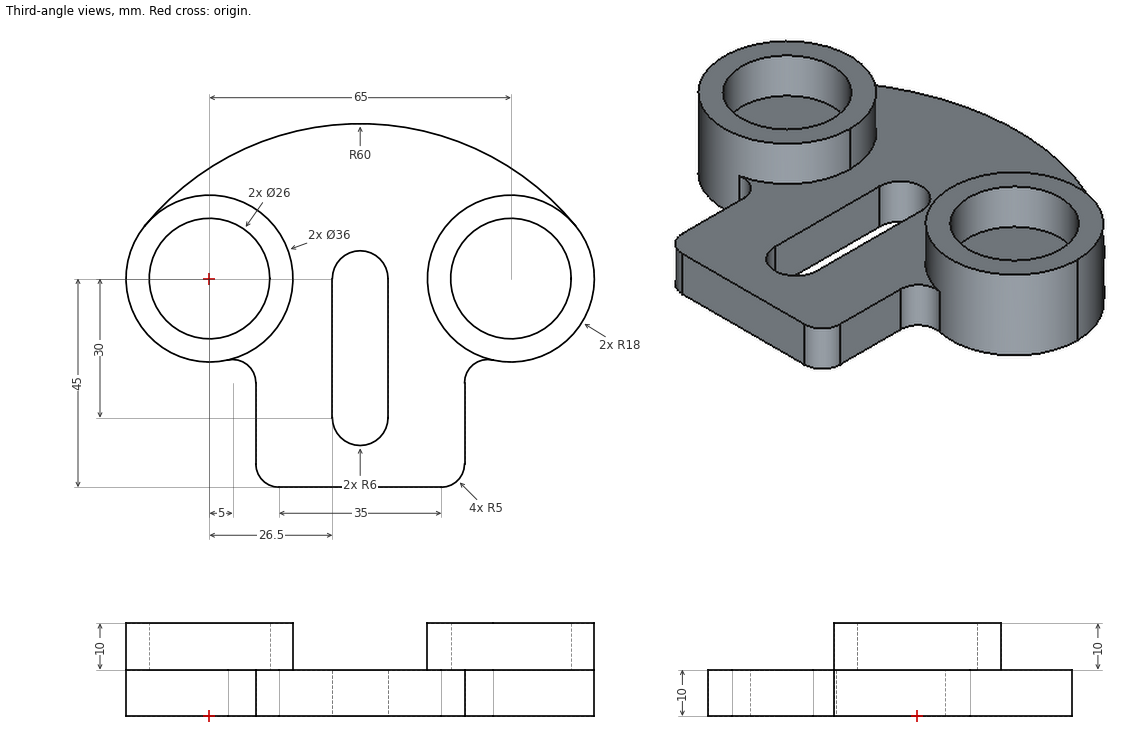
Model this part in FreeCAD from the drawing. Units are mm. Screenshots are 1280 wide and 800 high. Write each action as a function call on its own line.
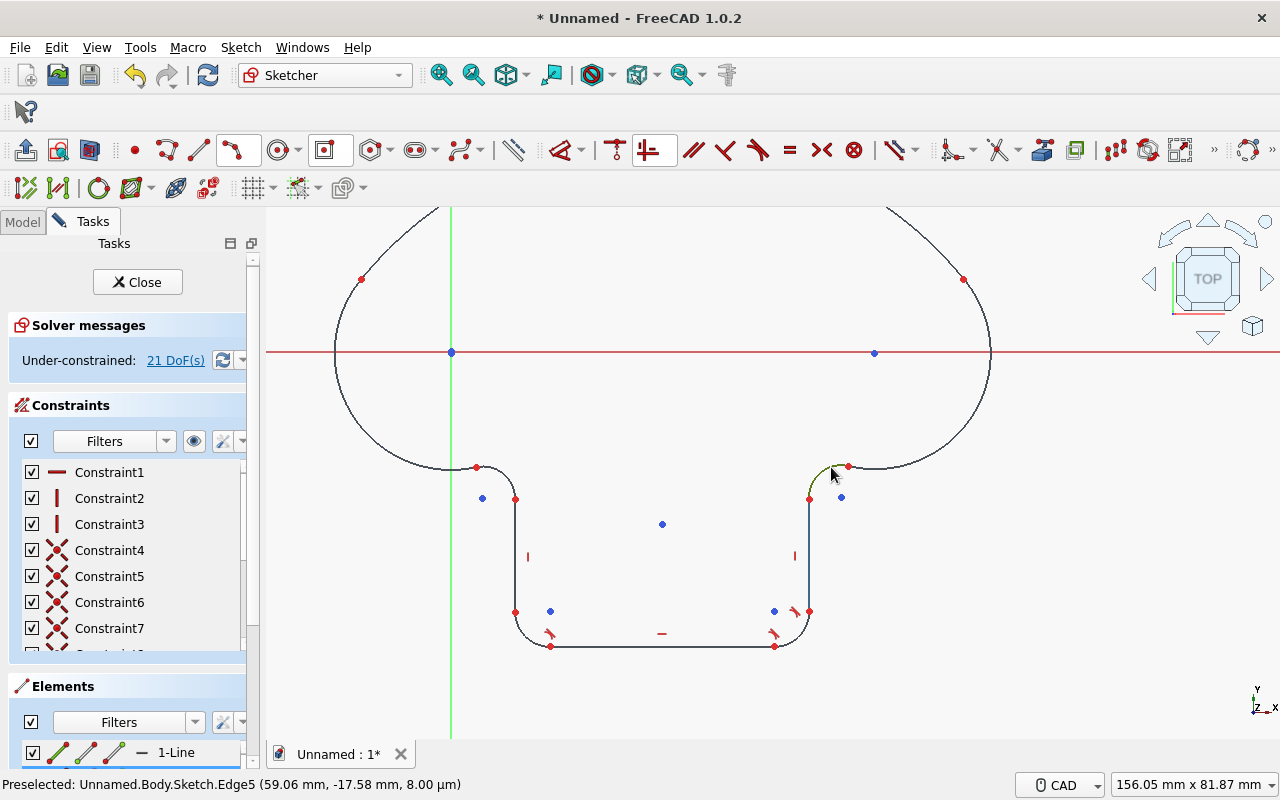
click(758, 150)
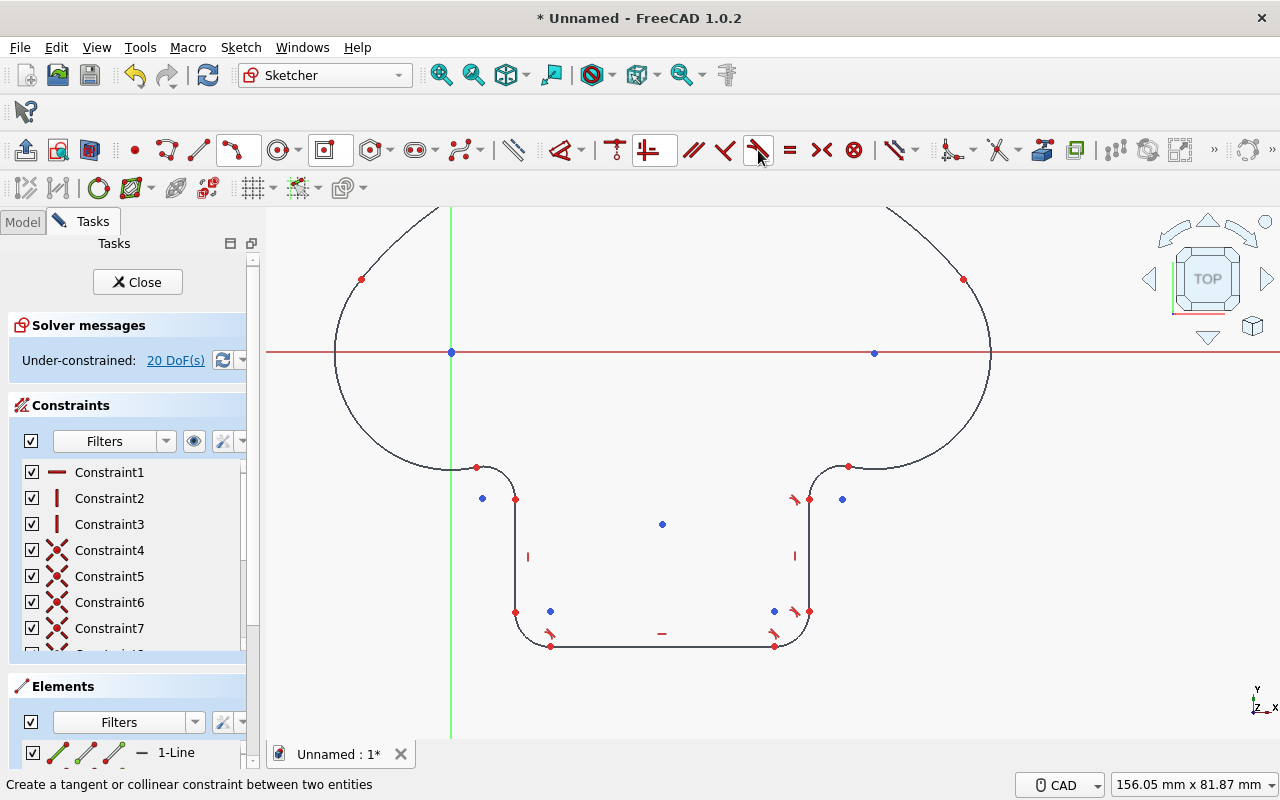
click(515, 534)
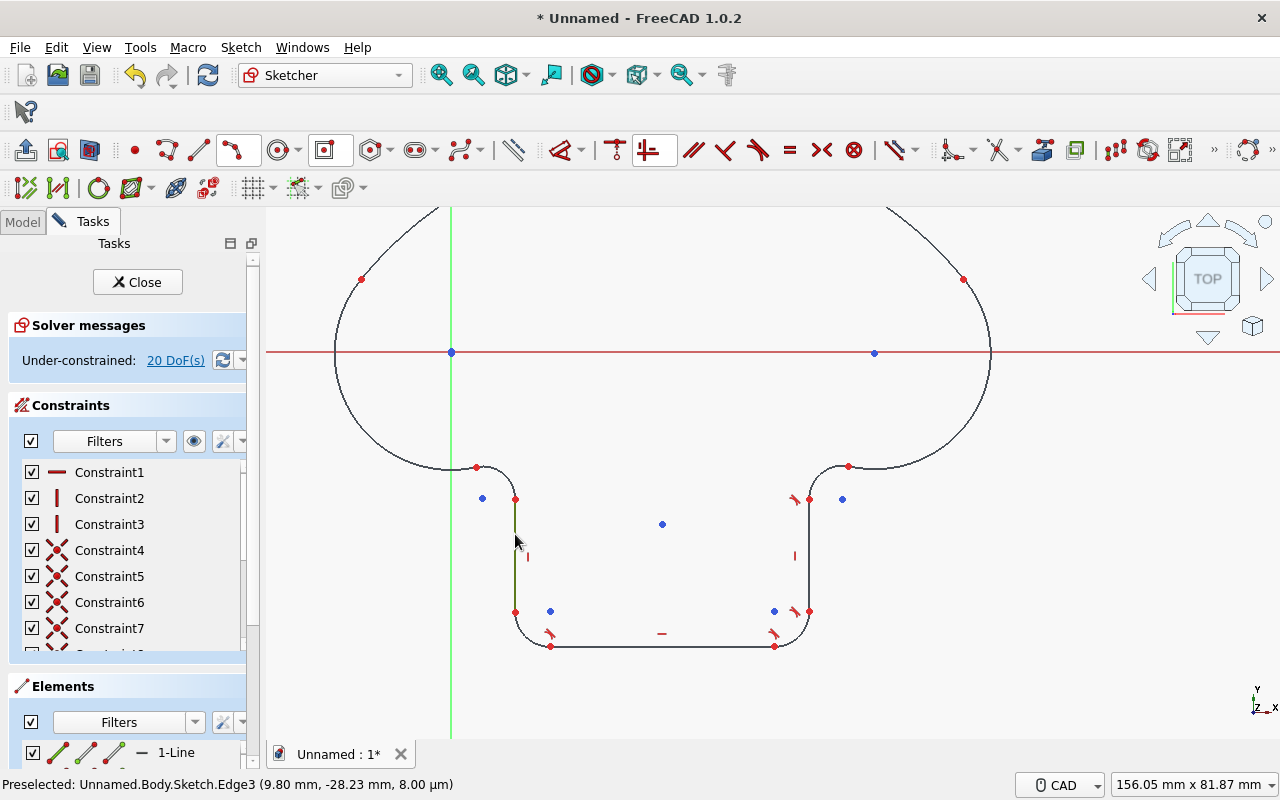
click(511, 483)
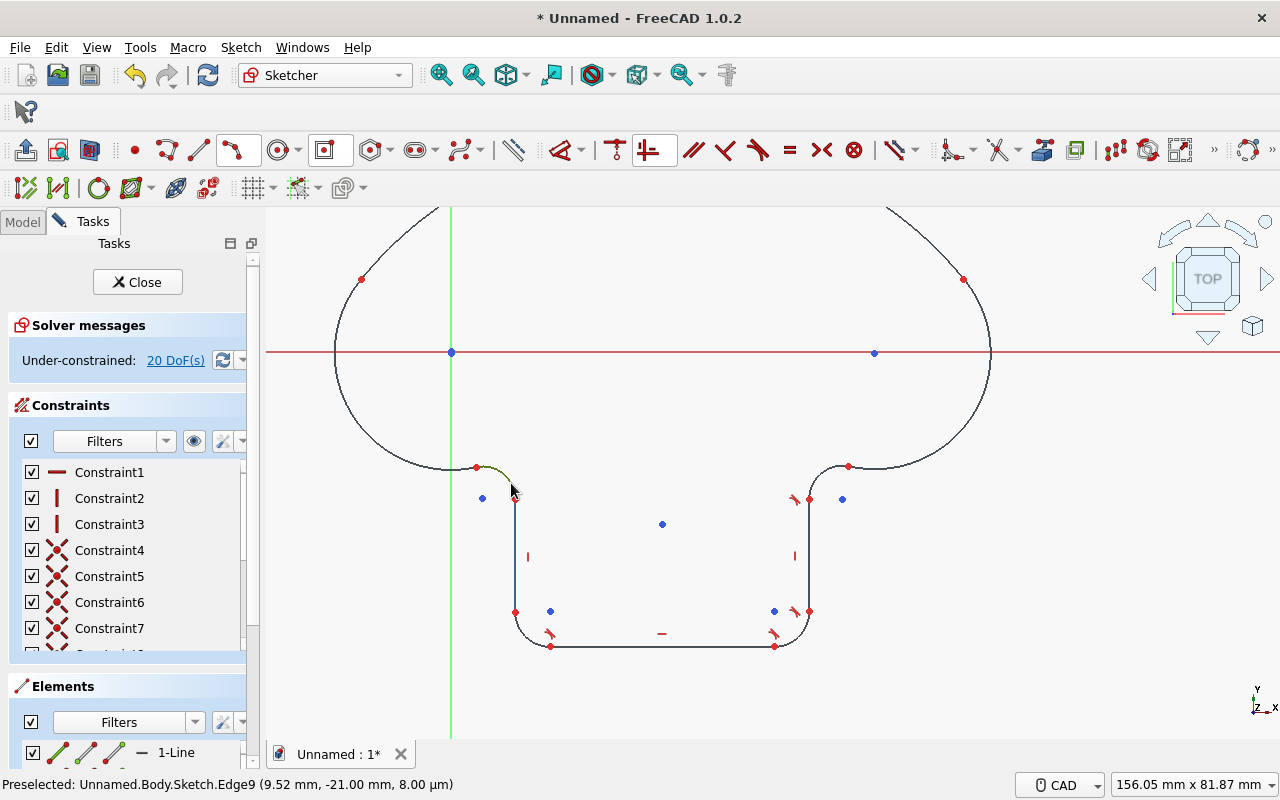
click(758, 150)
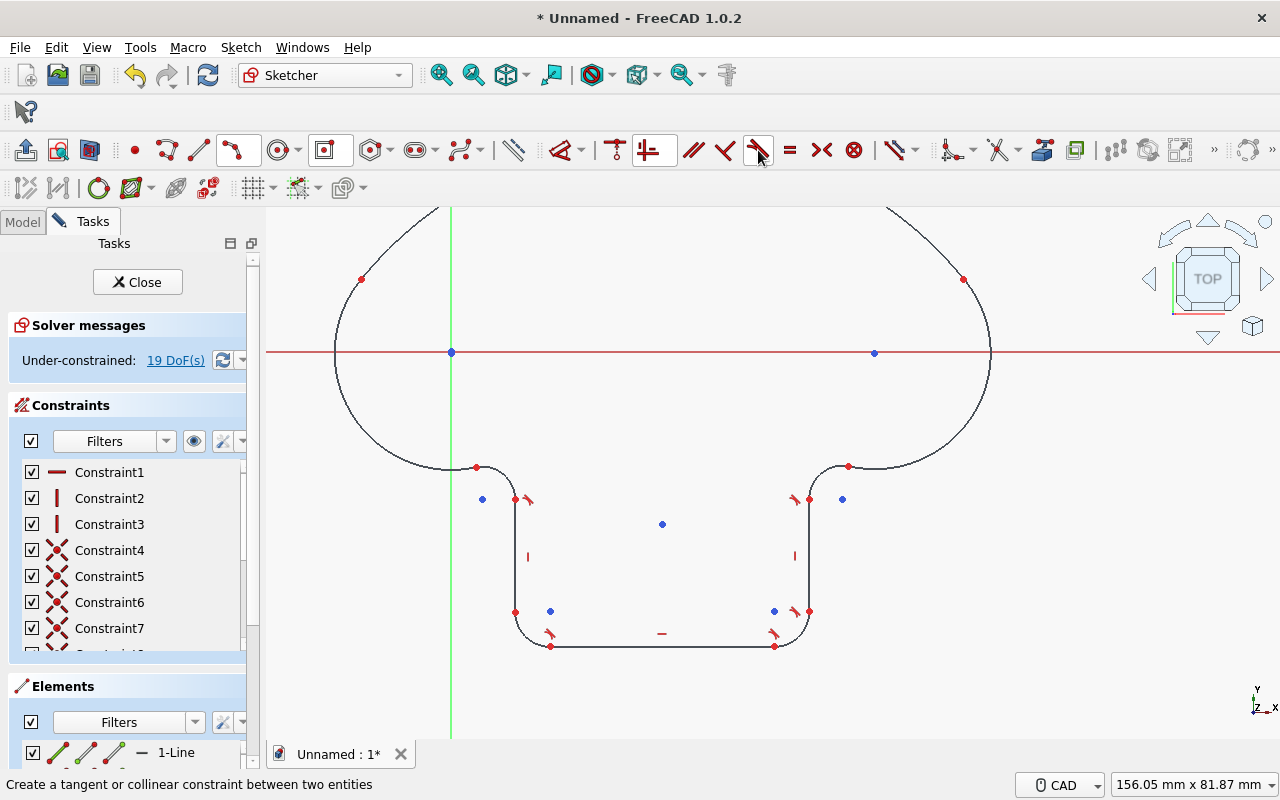
click(515, 534)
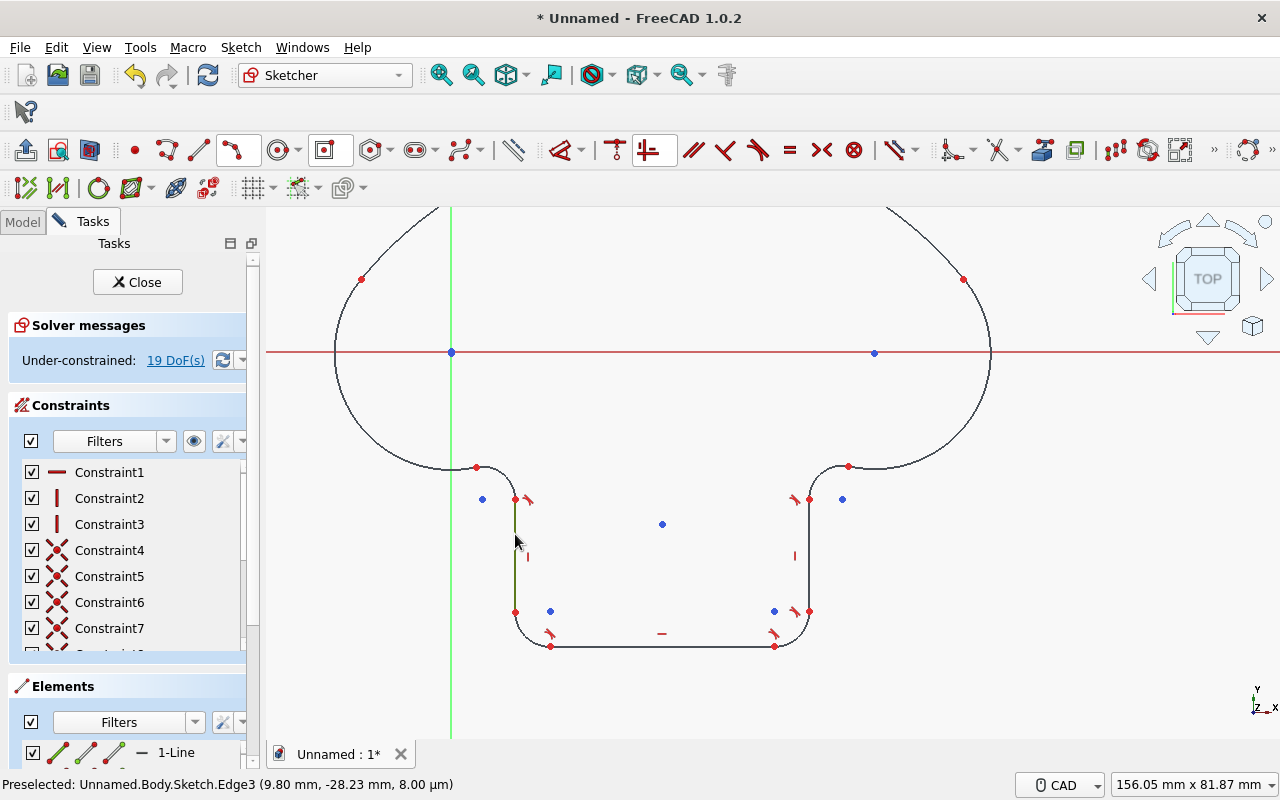
click(519, 628)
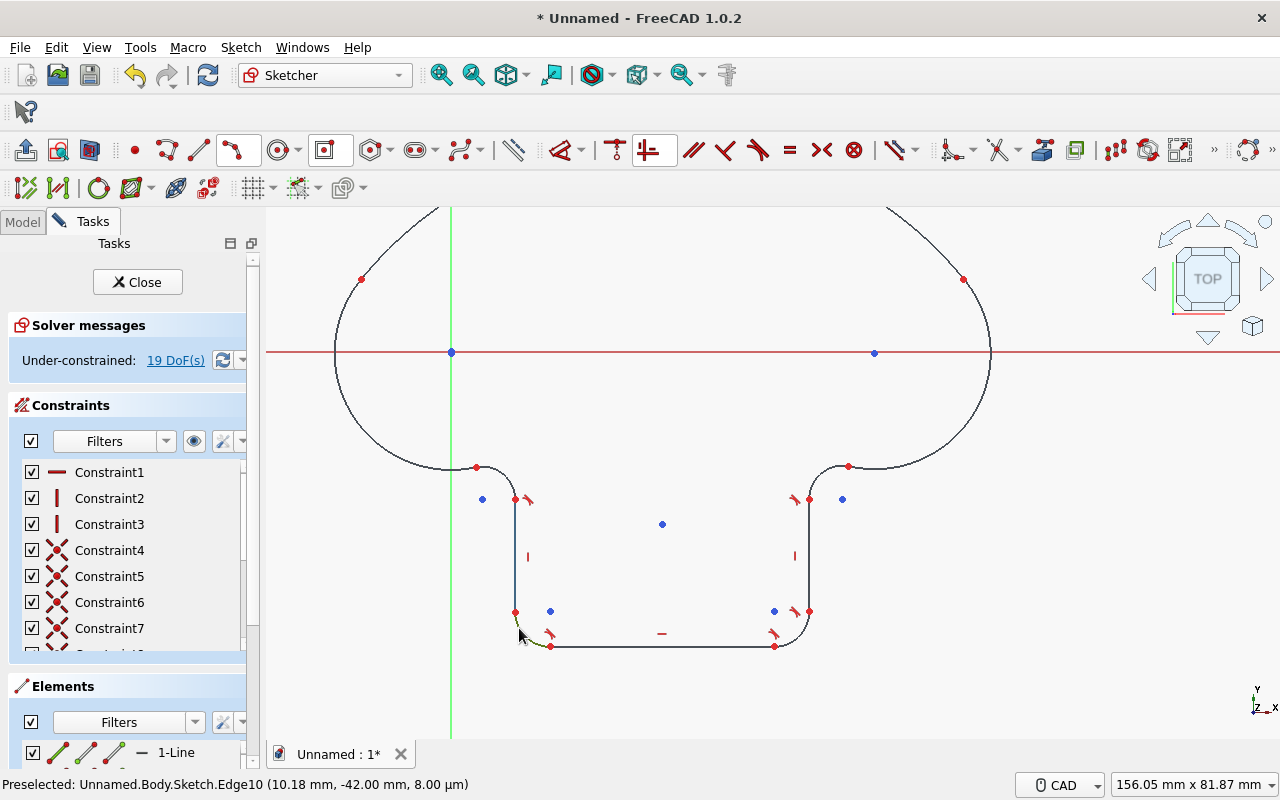
click(758, 150)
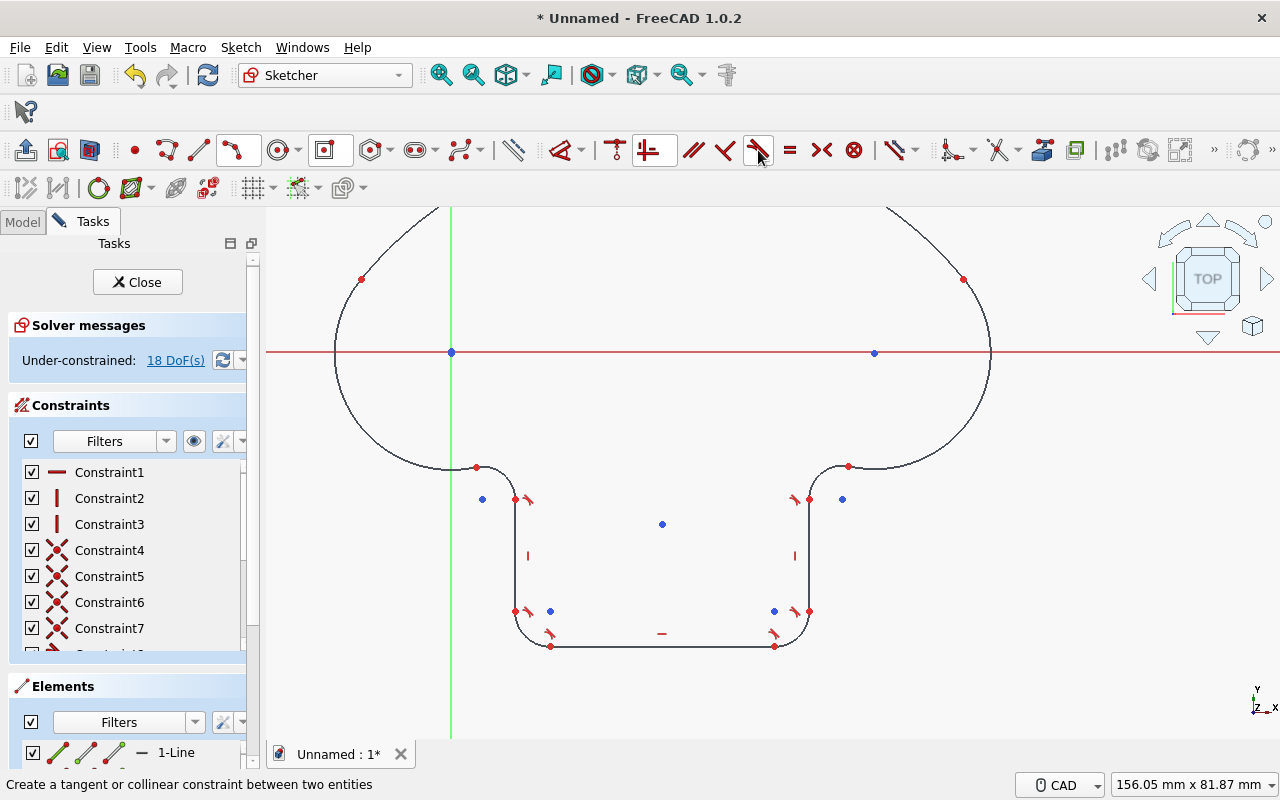
click(831, 468)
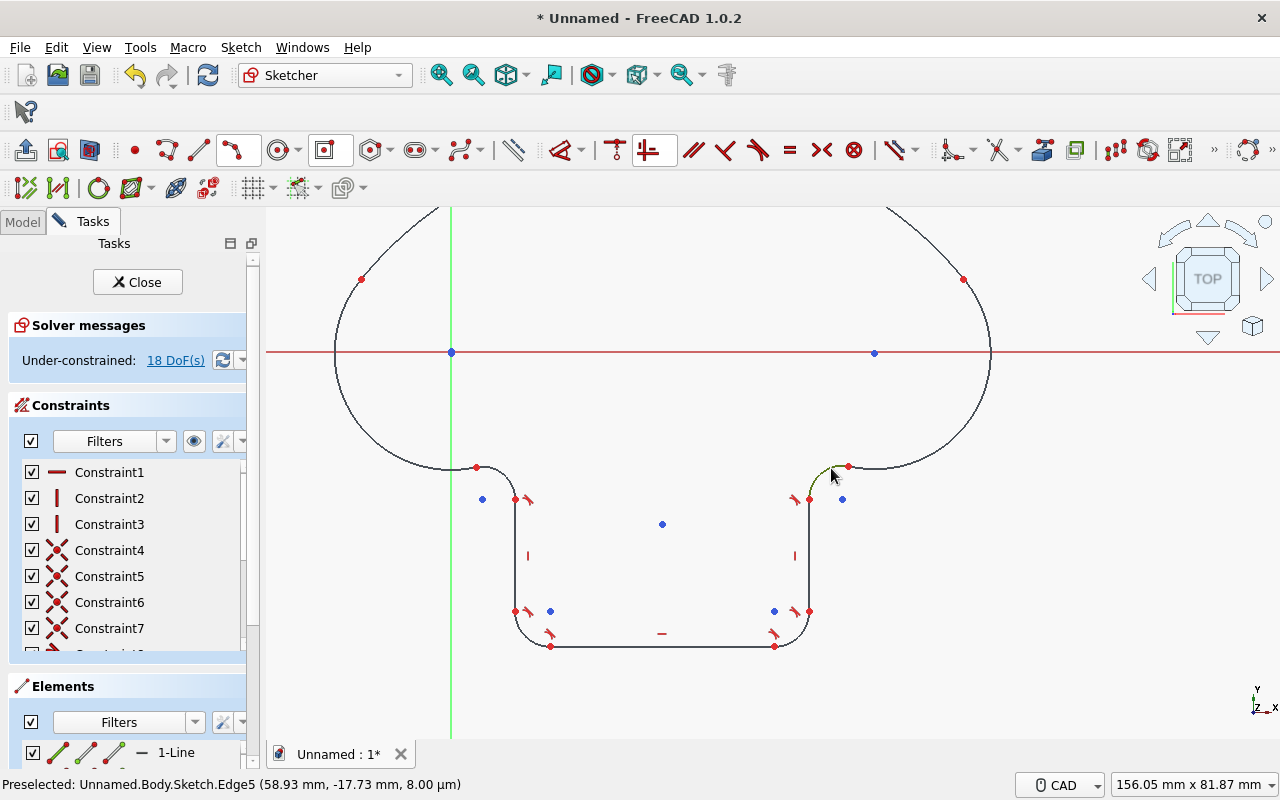
click(932, 454)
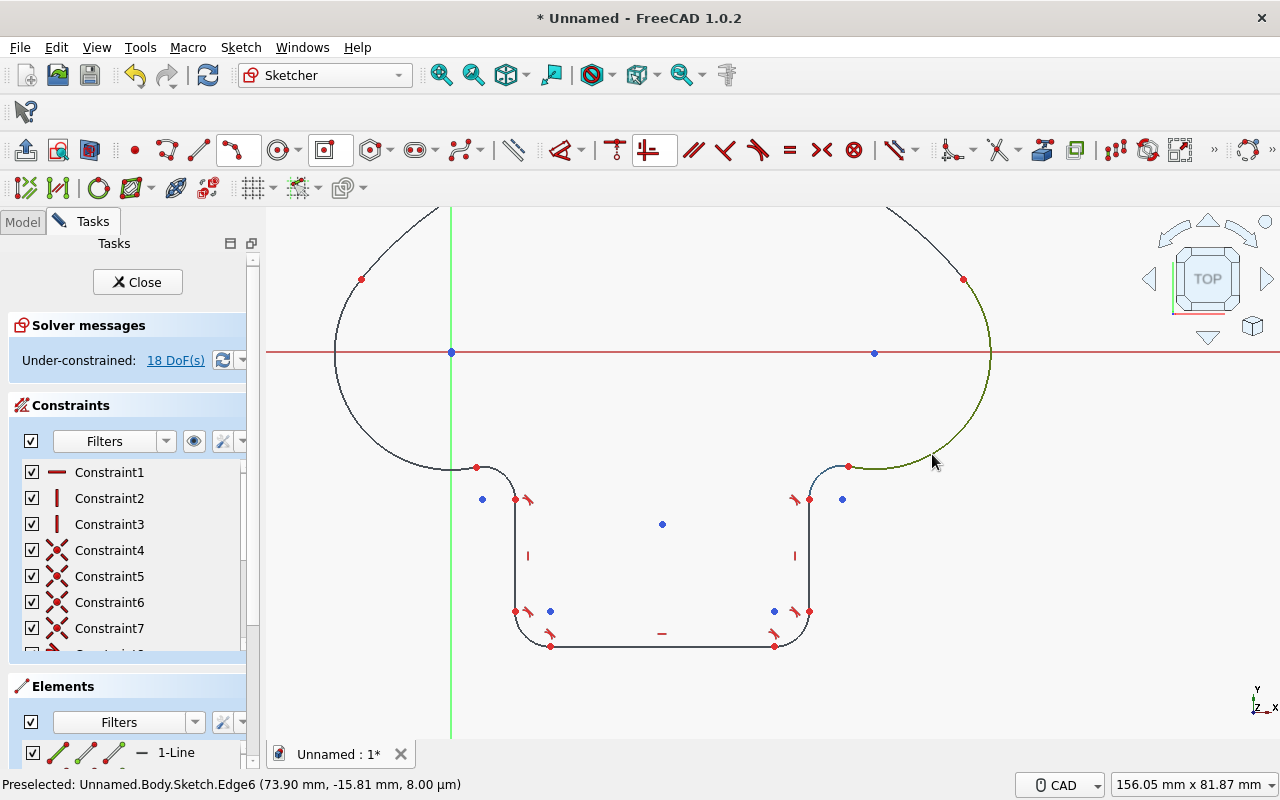
click(758, 150)